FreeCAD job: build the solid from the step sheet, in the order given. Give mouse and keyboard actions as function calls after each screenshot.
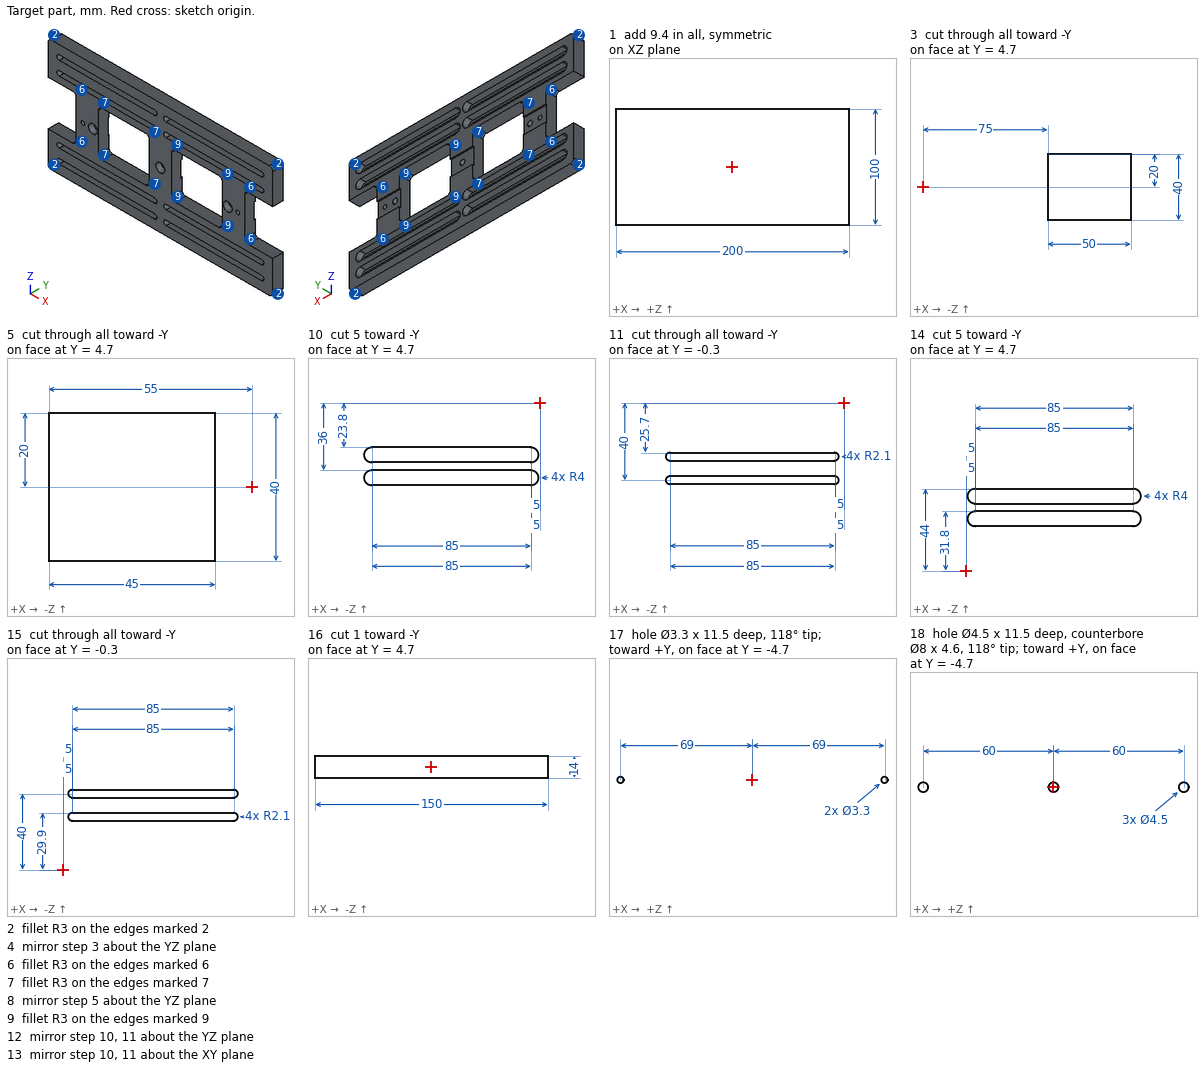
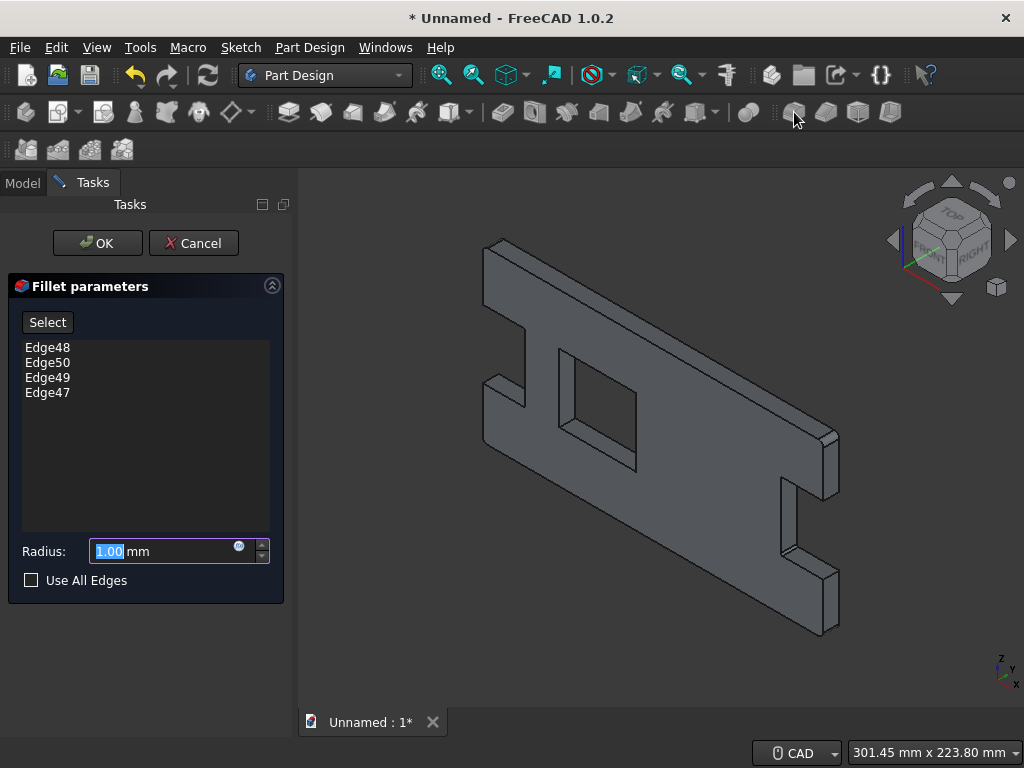
text(3)
key(Tab)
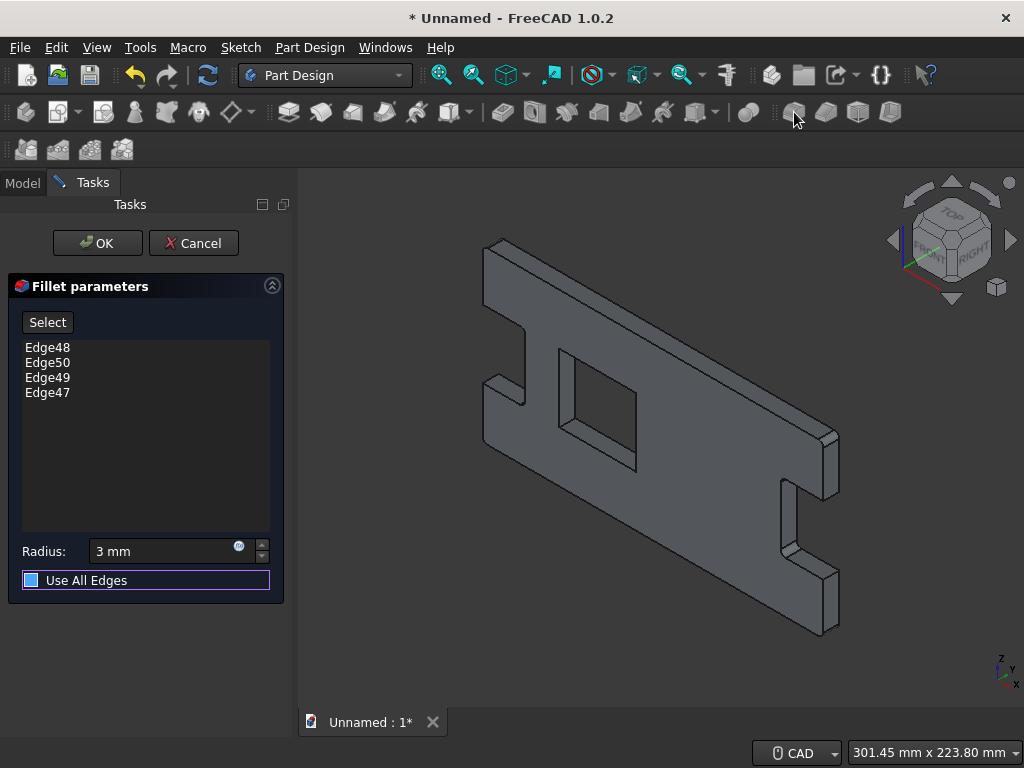
click(98, 243)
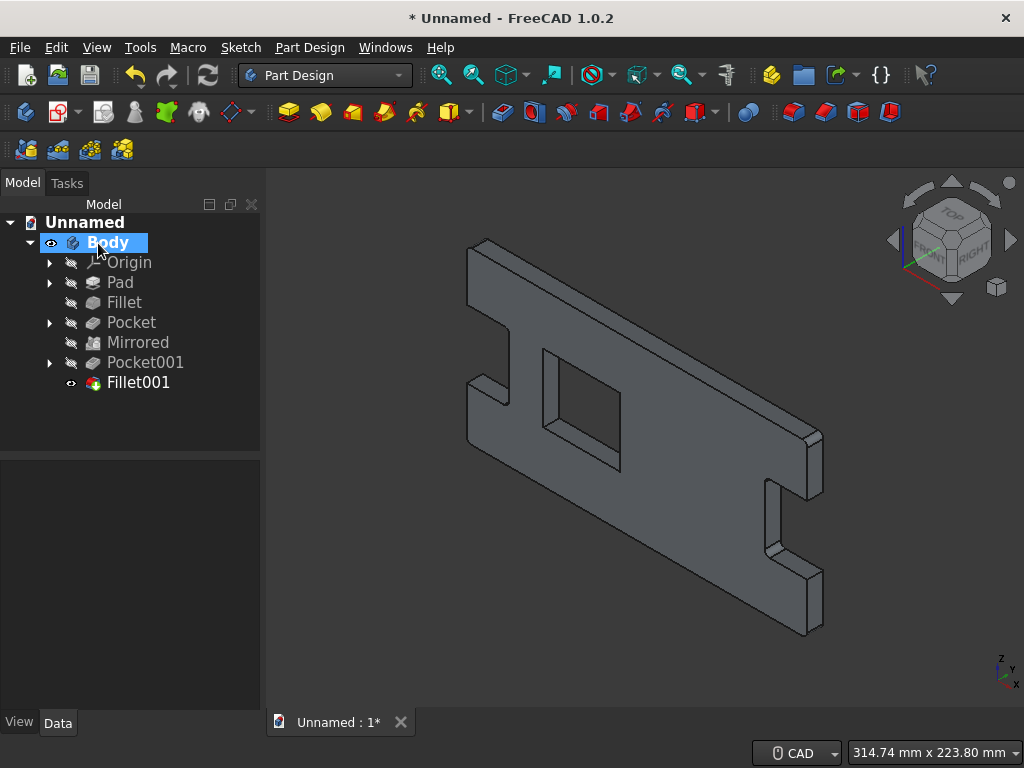
key(2)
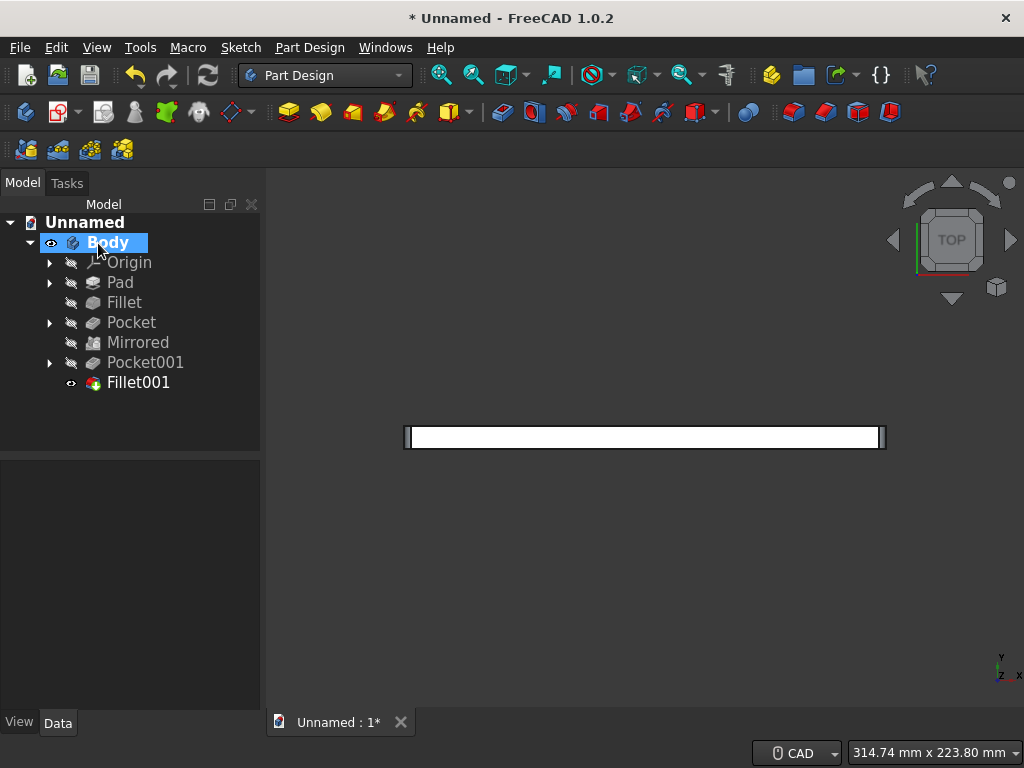
key(0)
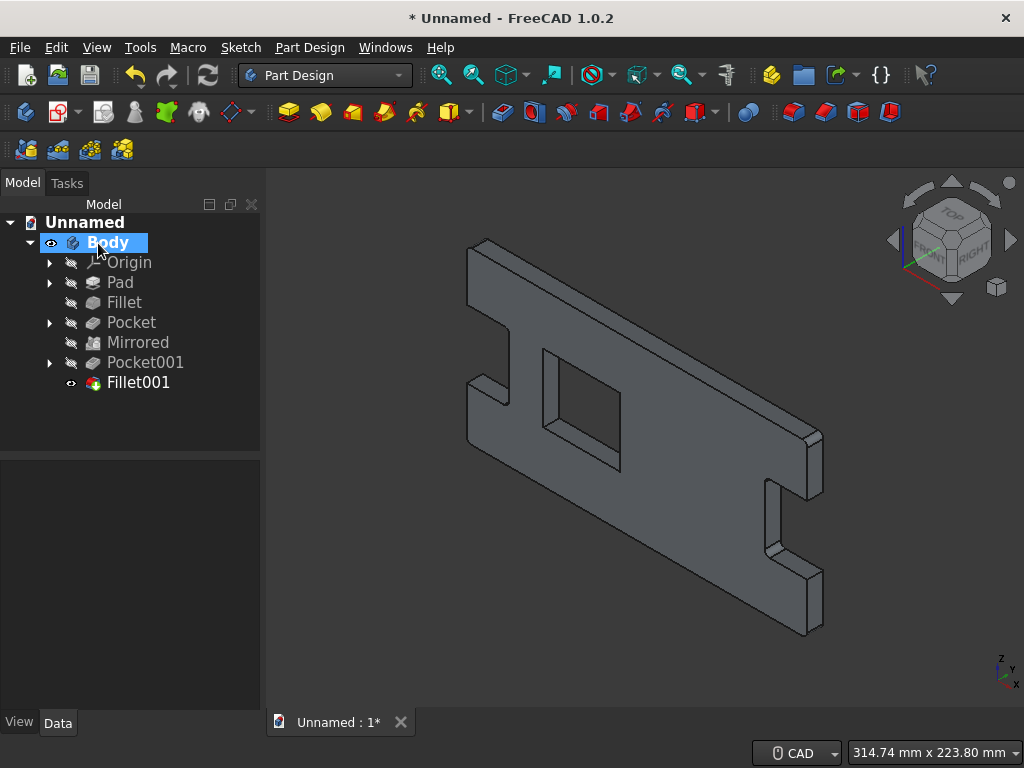
key(1)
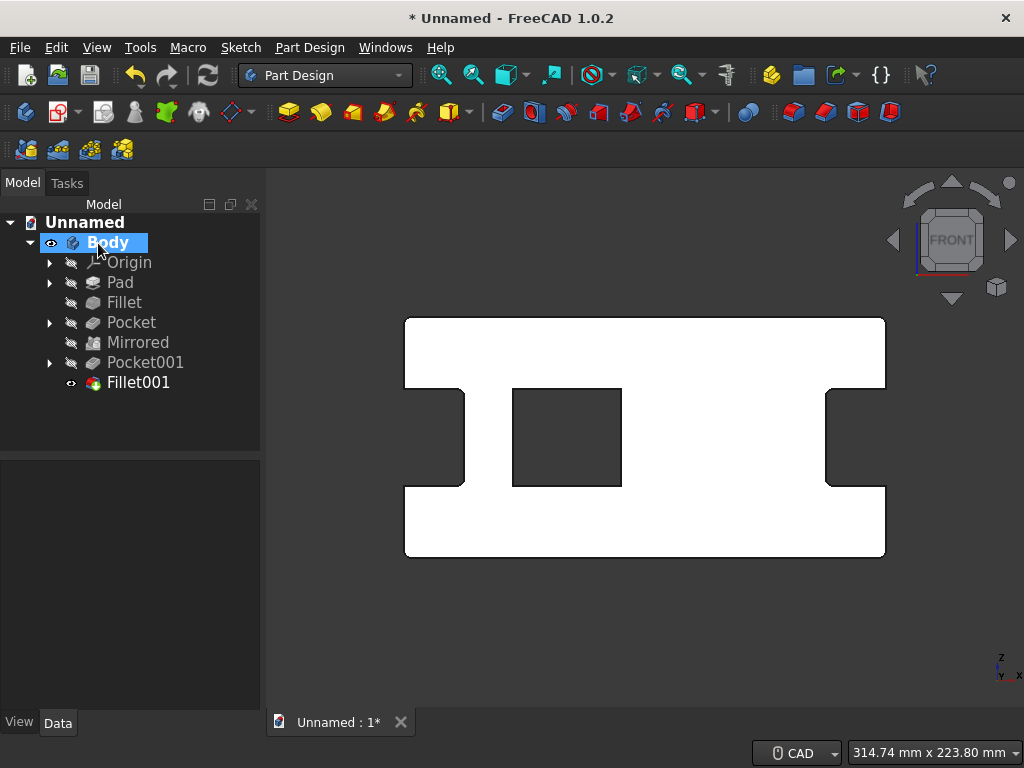
key(3)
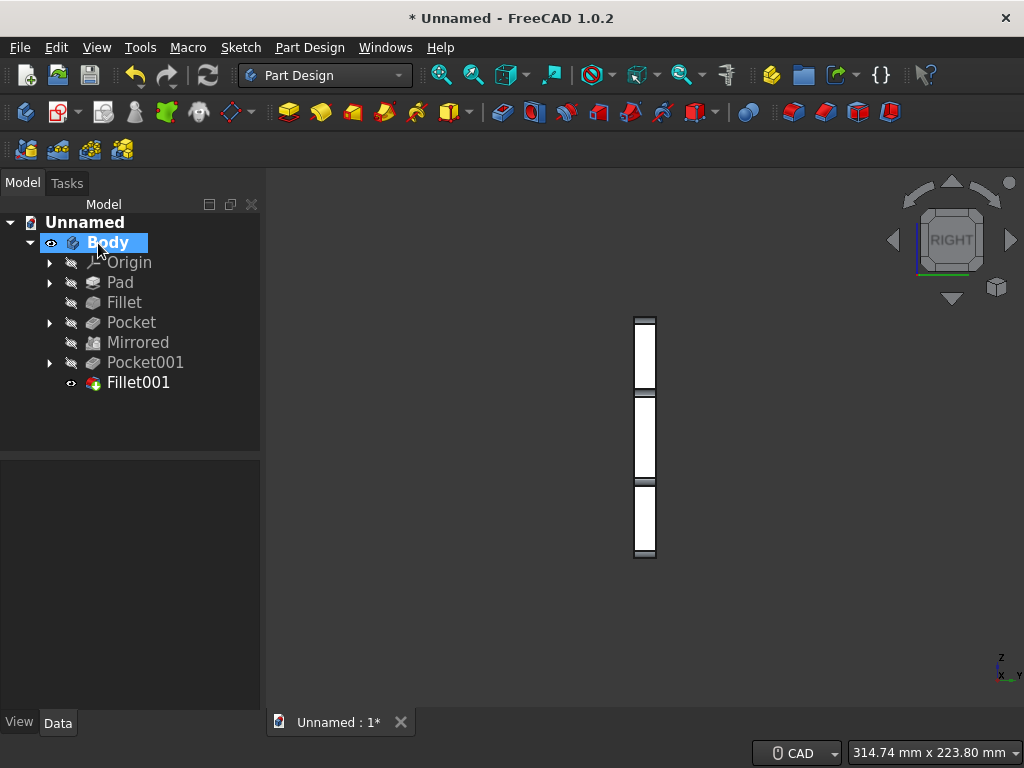
key(v)
key(f)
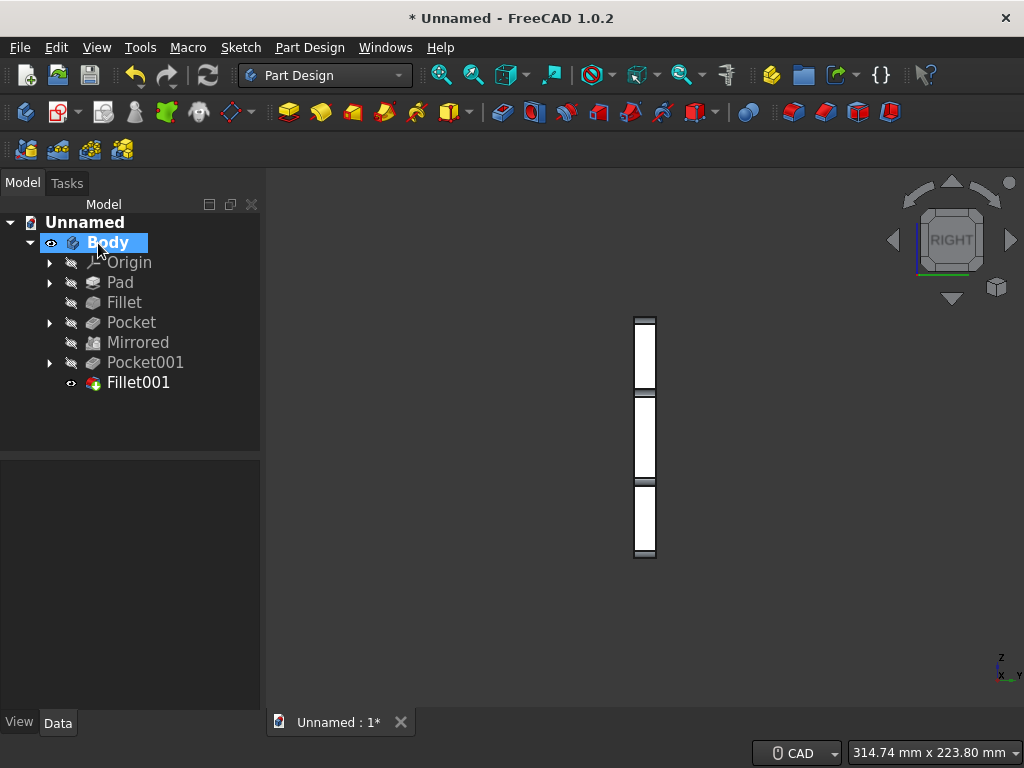
key(5)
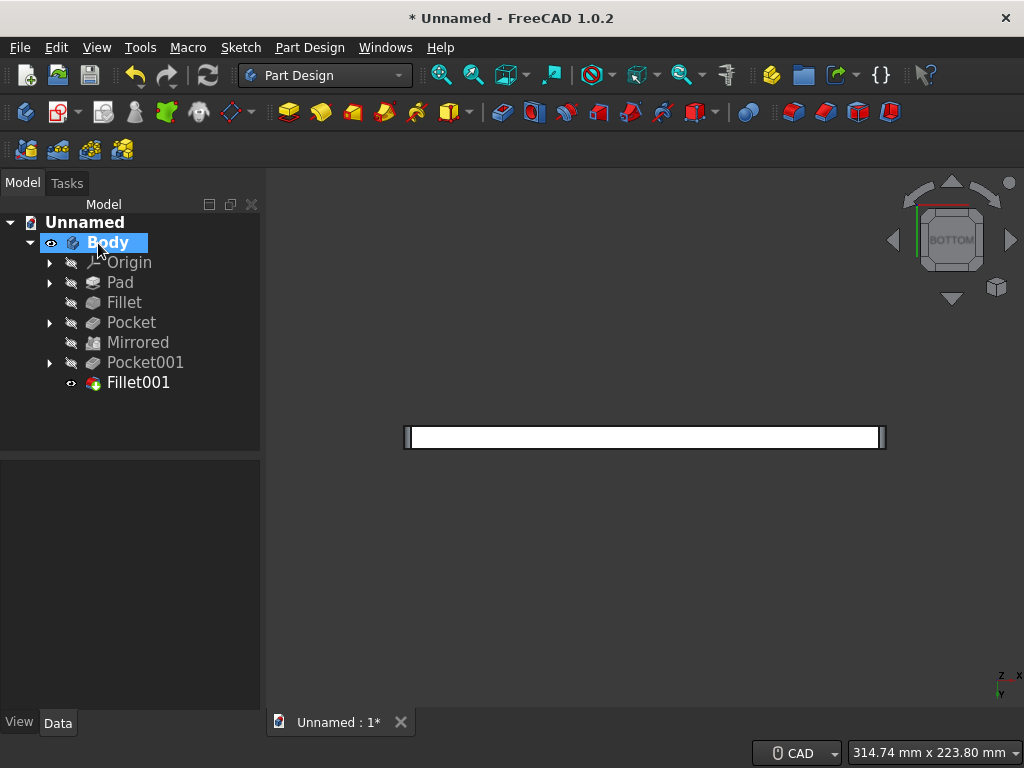
key(4)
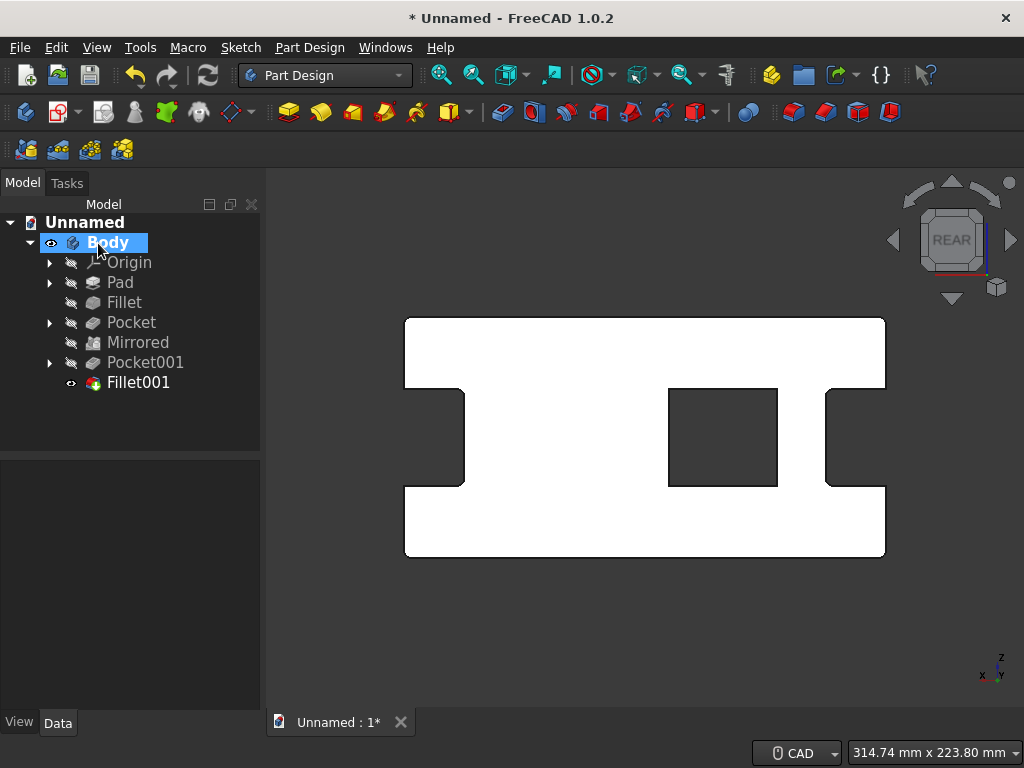
key(6)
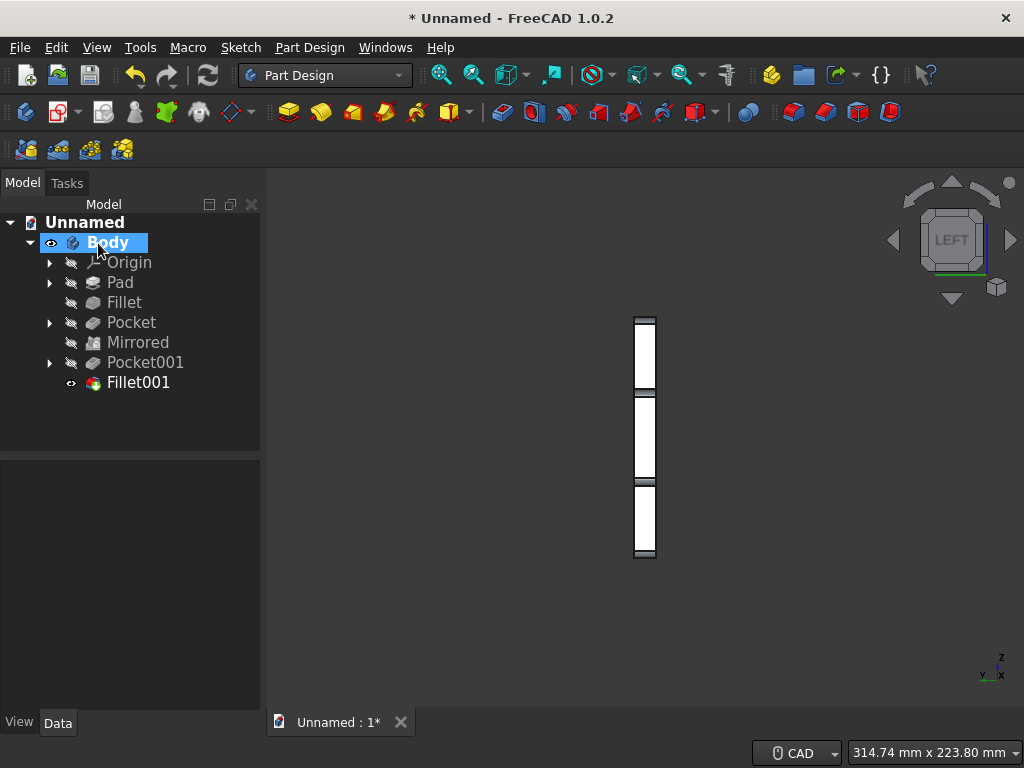
key(v)
key(f)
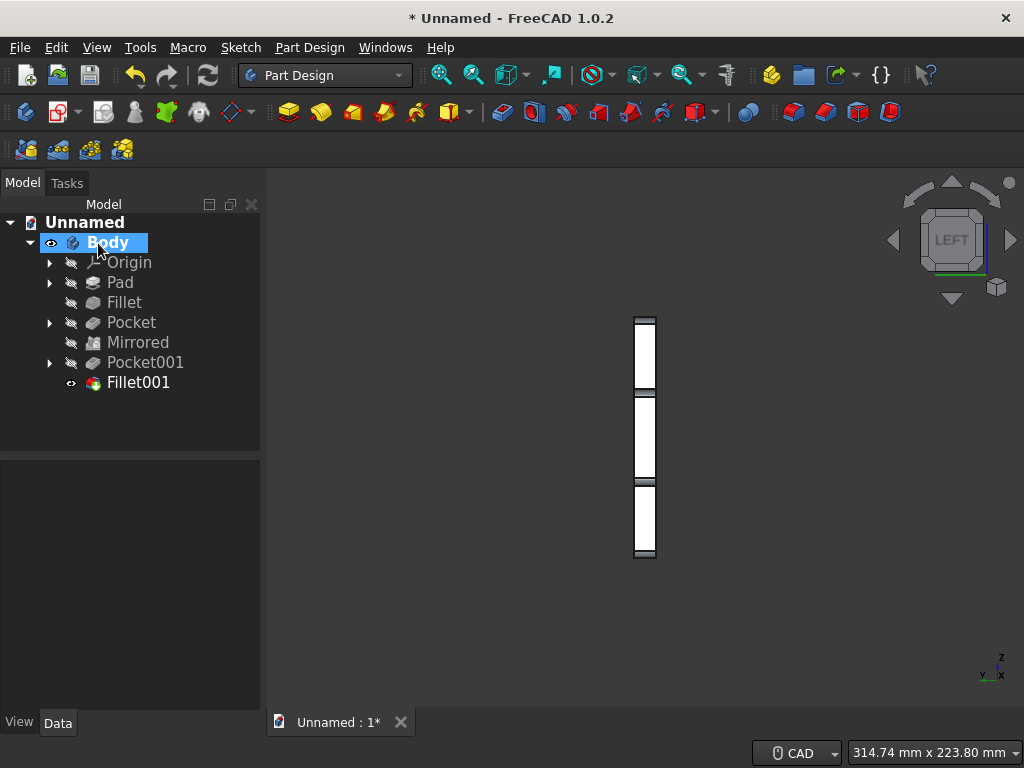
key(v)
key(3)